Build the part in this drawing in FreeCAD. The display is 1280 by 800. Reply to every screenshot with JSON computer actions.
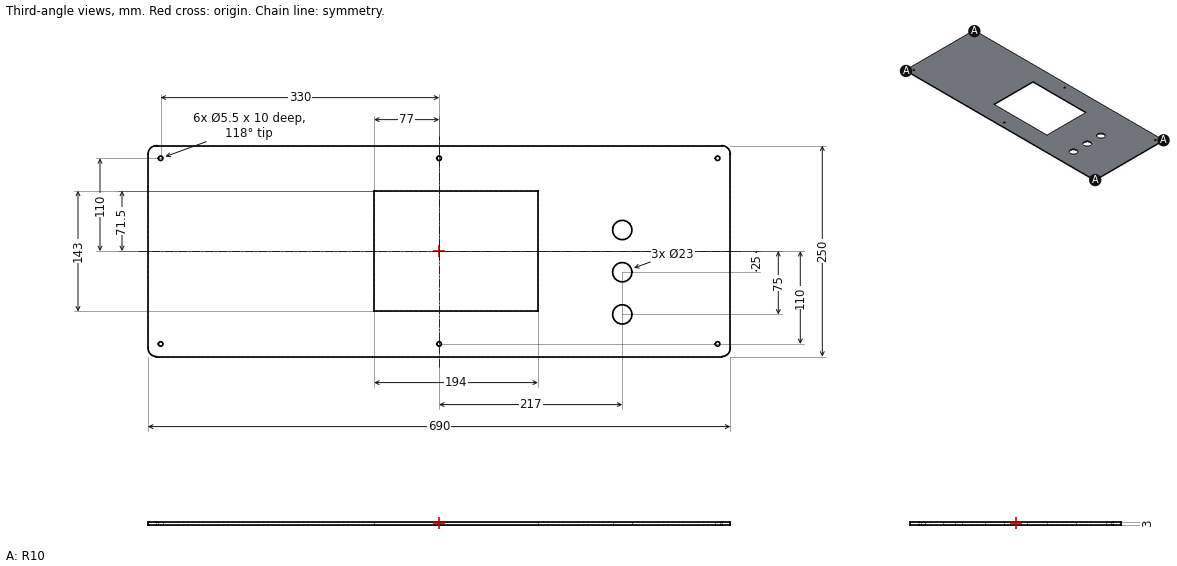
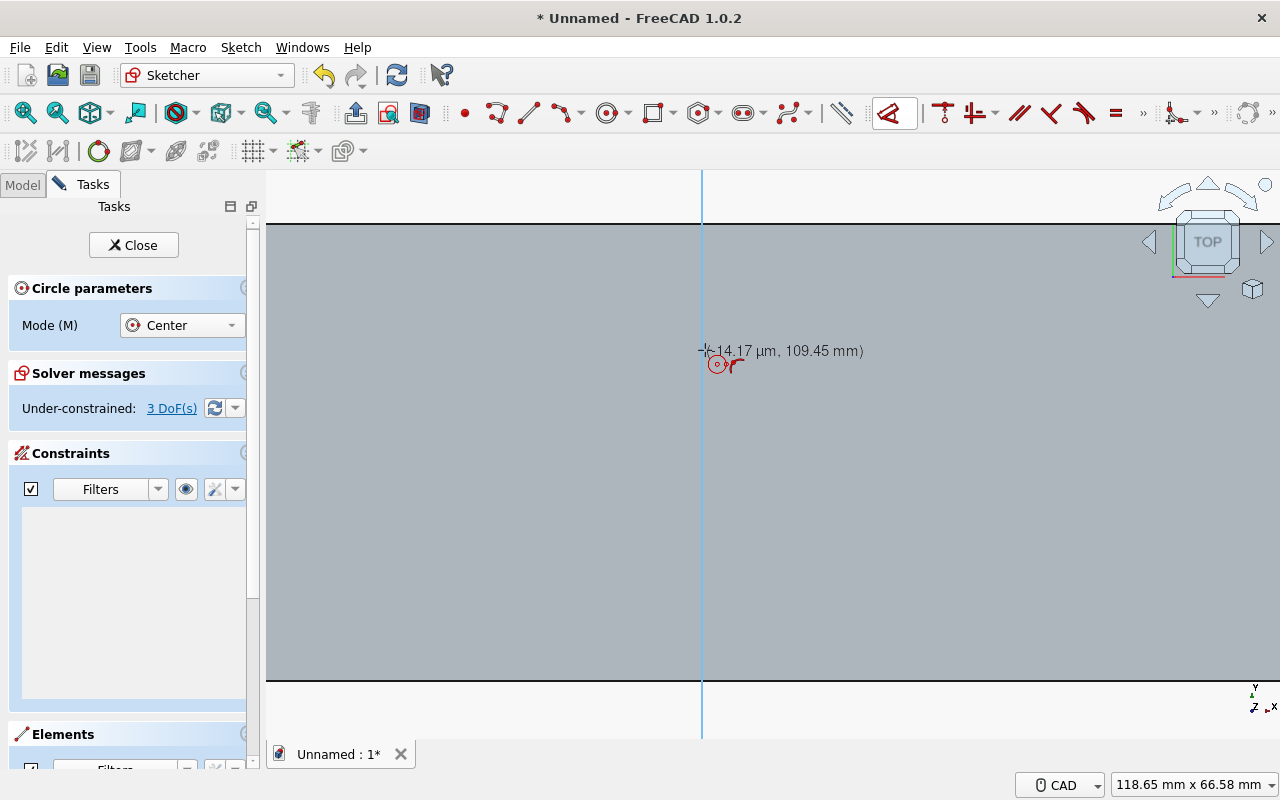
{"action": "scroll", "coordinate": [705, 350], "scroll_direction": "down", "scroll_amount": 11}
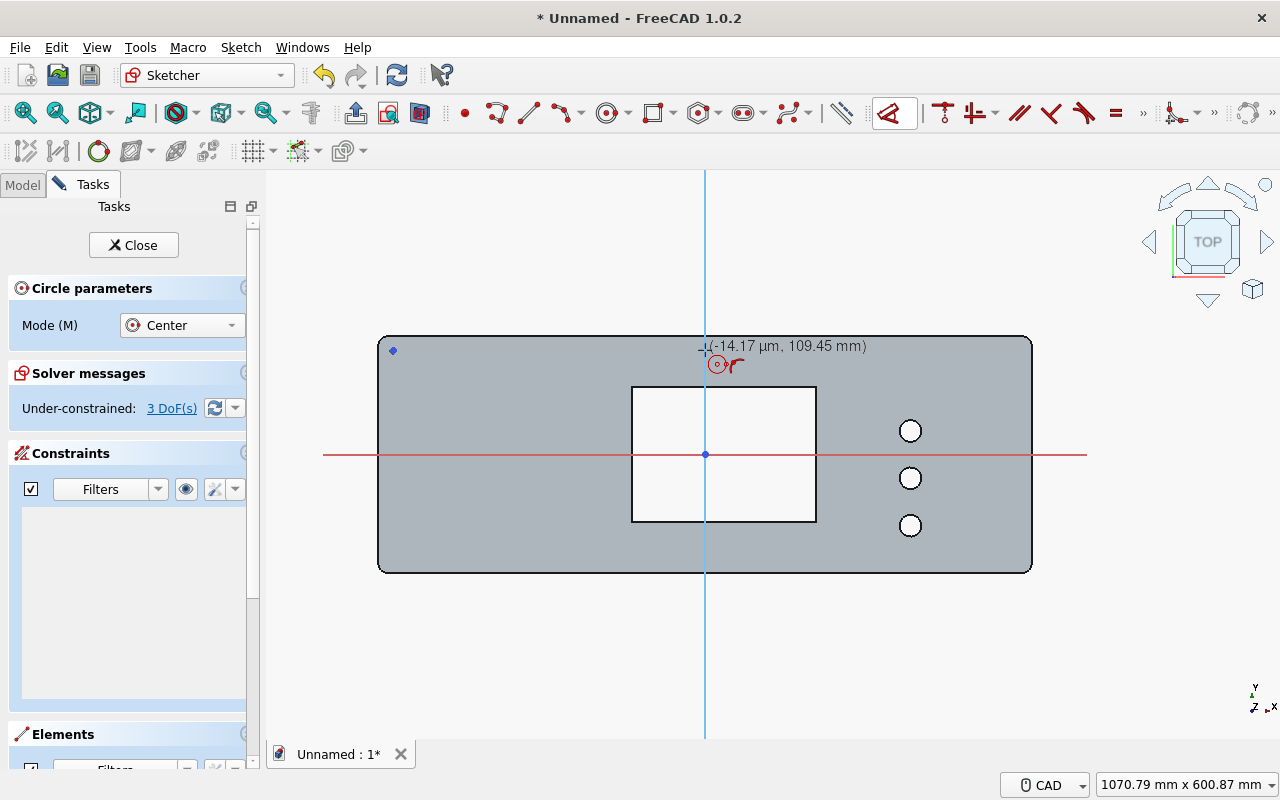
{"action": "left_click", "coordinate": [705, 350]}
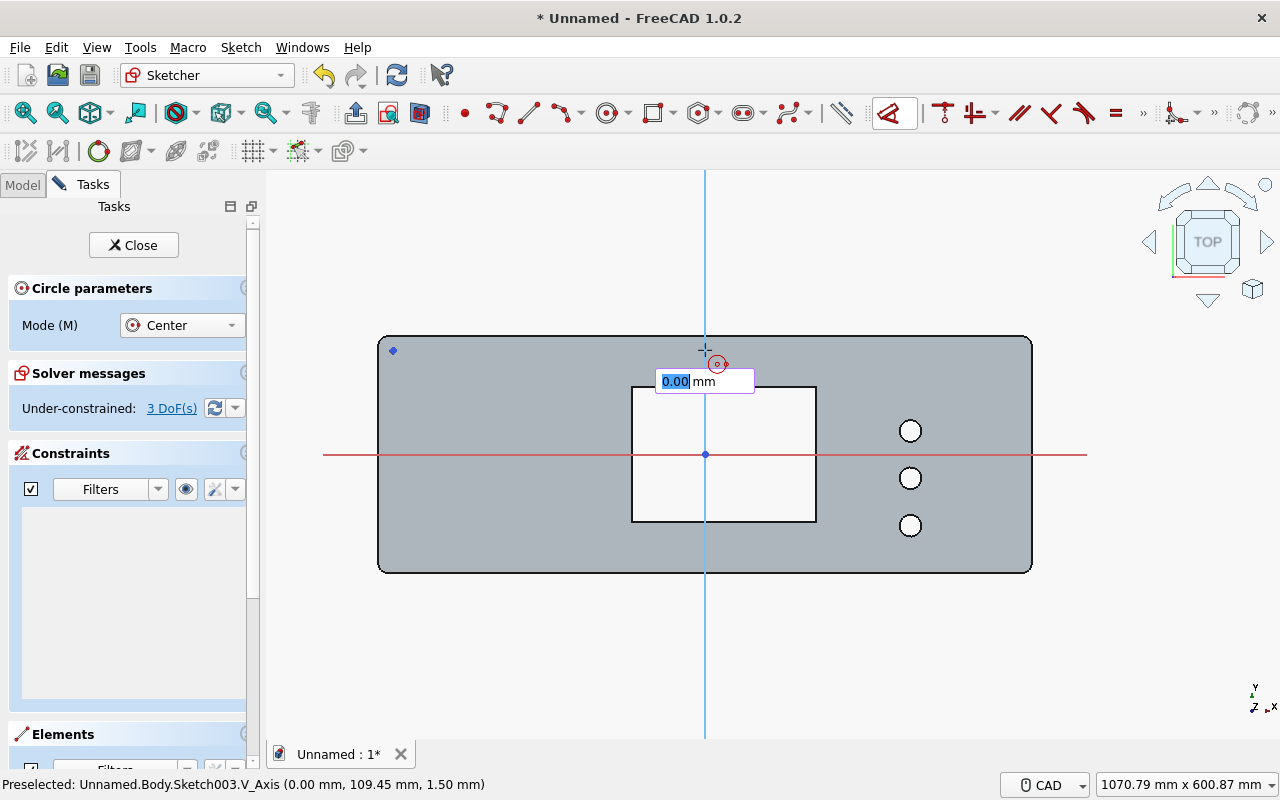
{"action": "scroll", "coordinate": [707, 350], "scroll_direction": "up", "scroll_amount": 10}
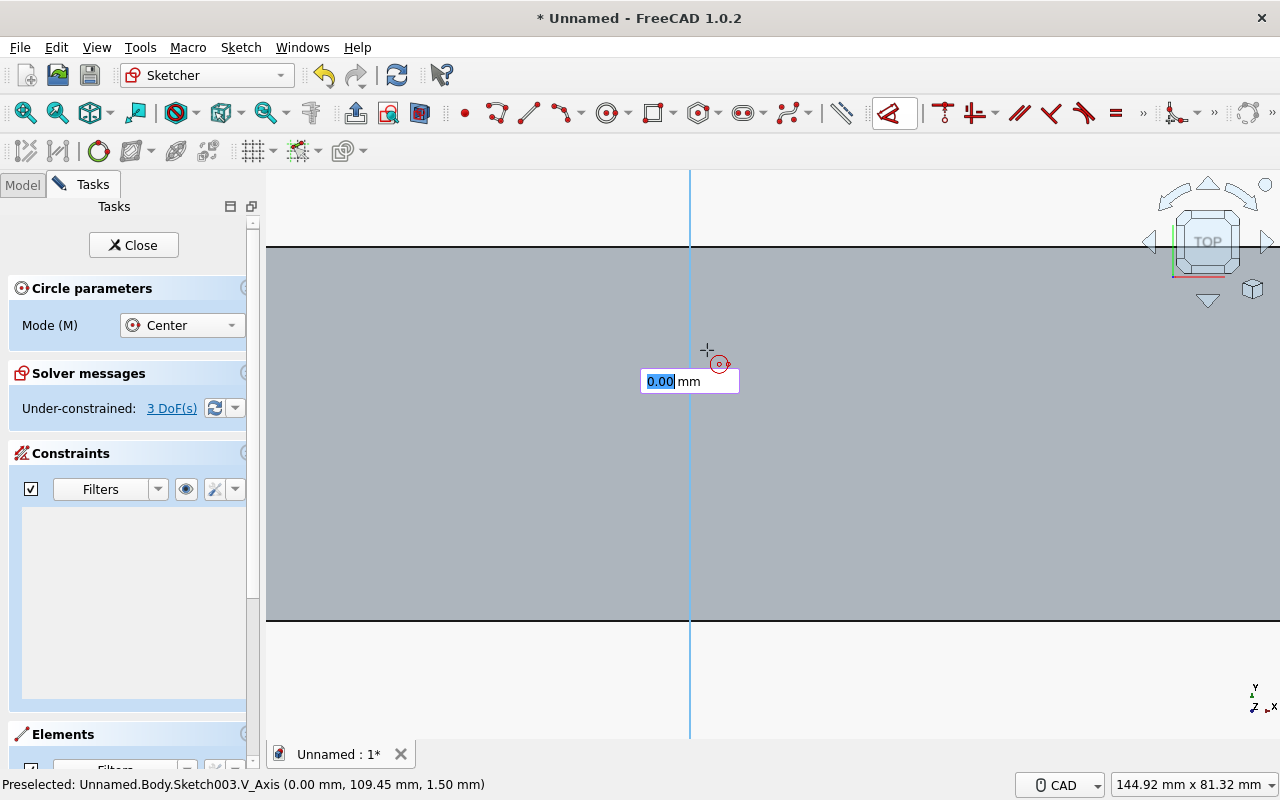
{"action": "left_click", "coordinate": [708, 345]}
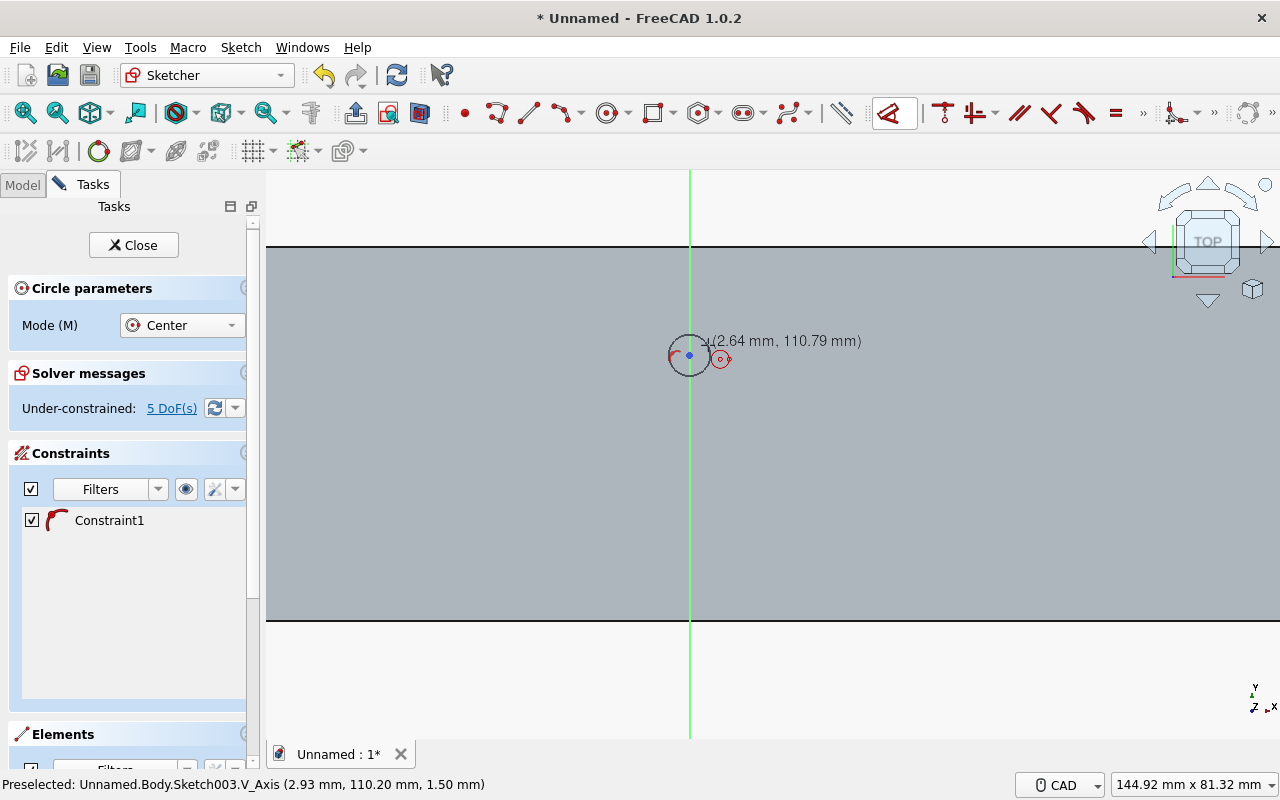
{"action": "scroll", "coordinate": [707, 350], "scroll_direction": "down", "scroll_amount": 10}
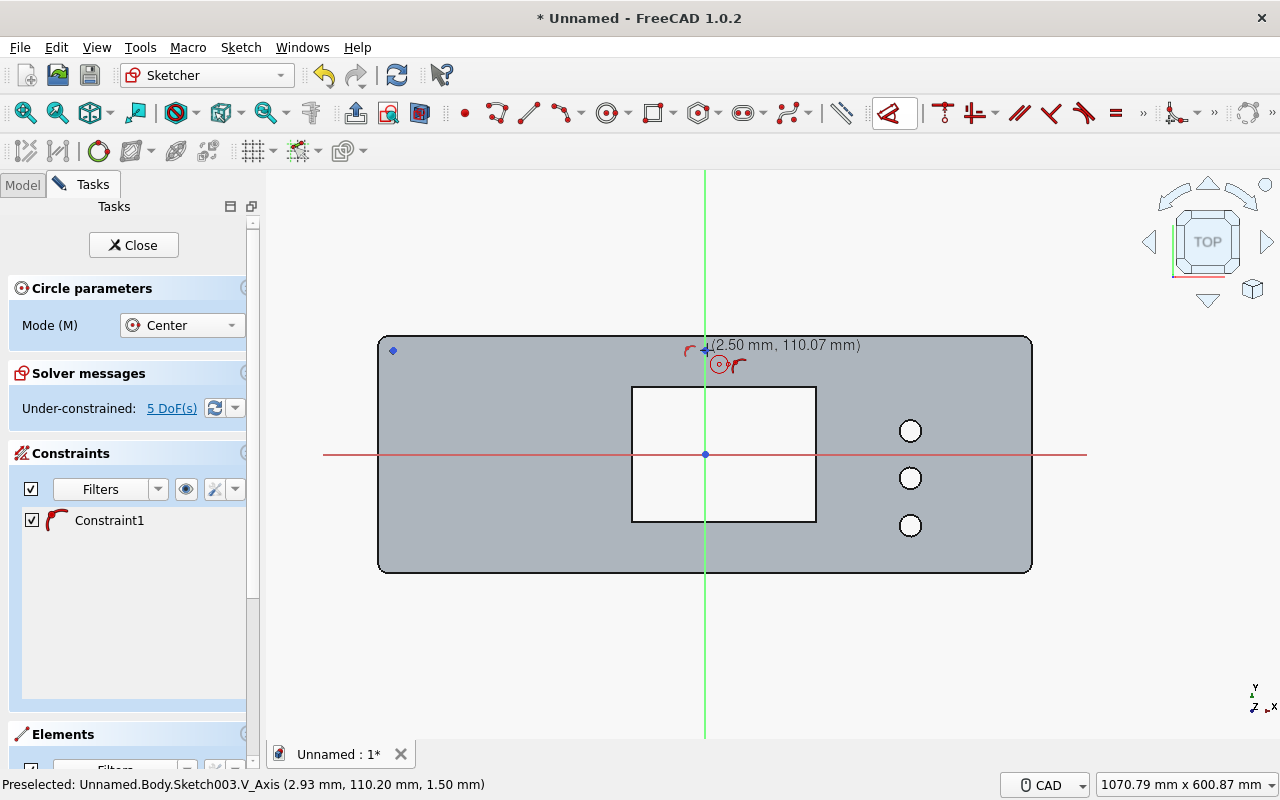
{"action": "scroll", "coordinate": [1018, 350], "scroll_direction": "up", "scroll_amount": 11}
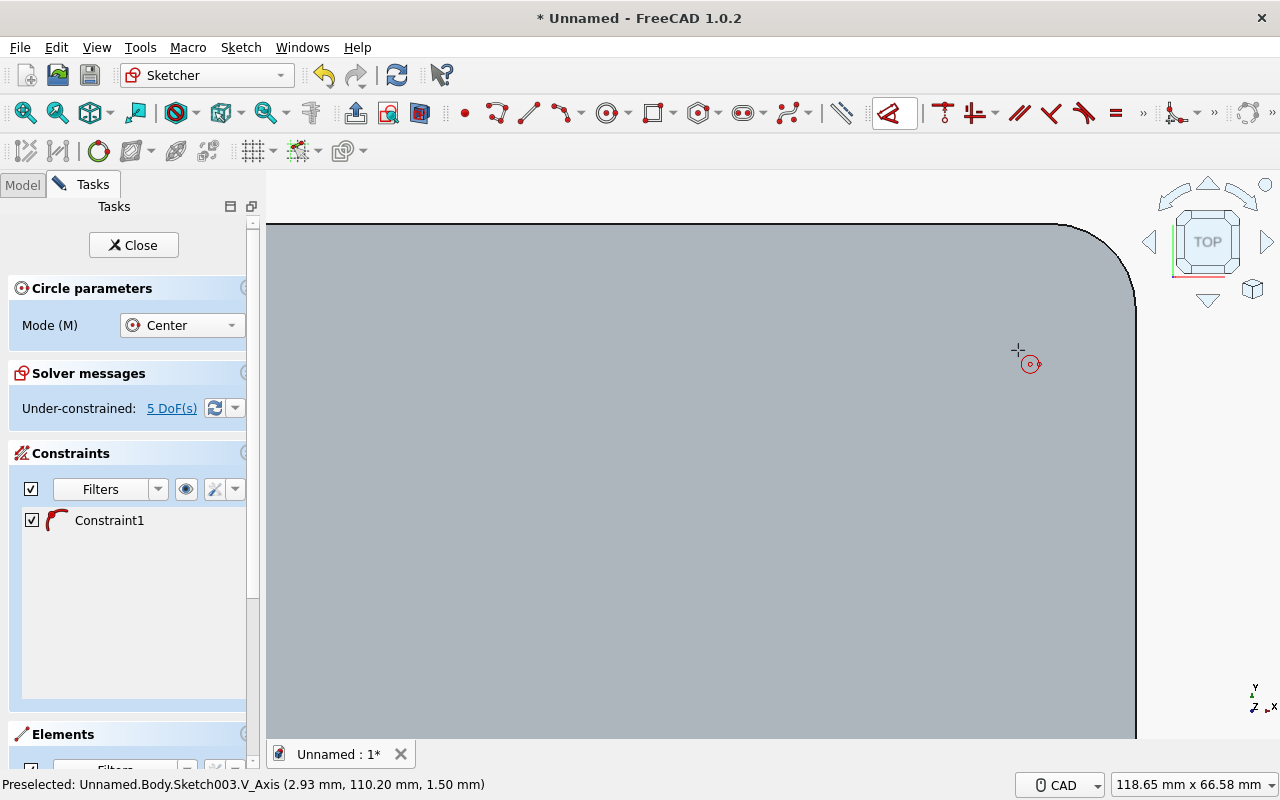
{"action": "scroll", "coordinate": [1018, 350], "scroll_direction": "down", "scroll_amount": 11}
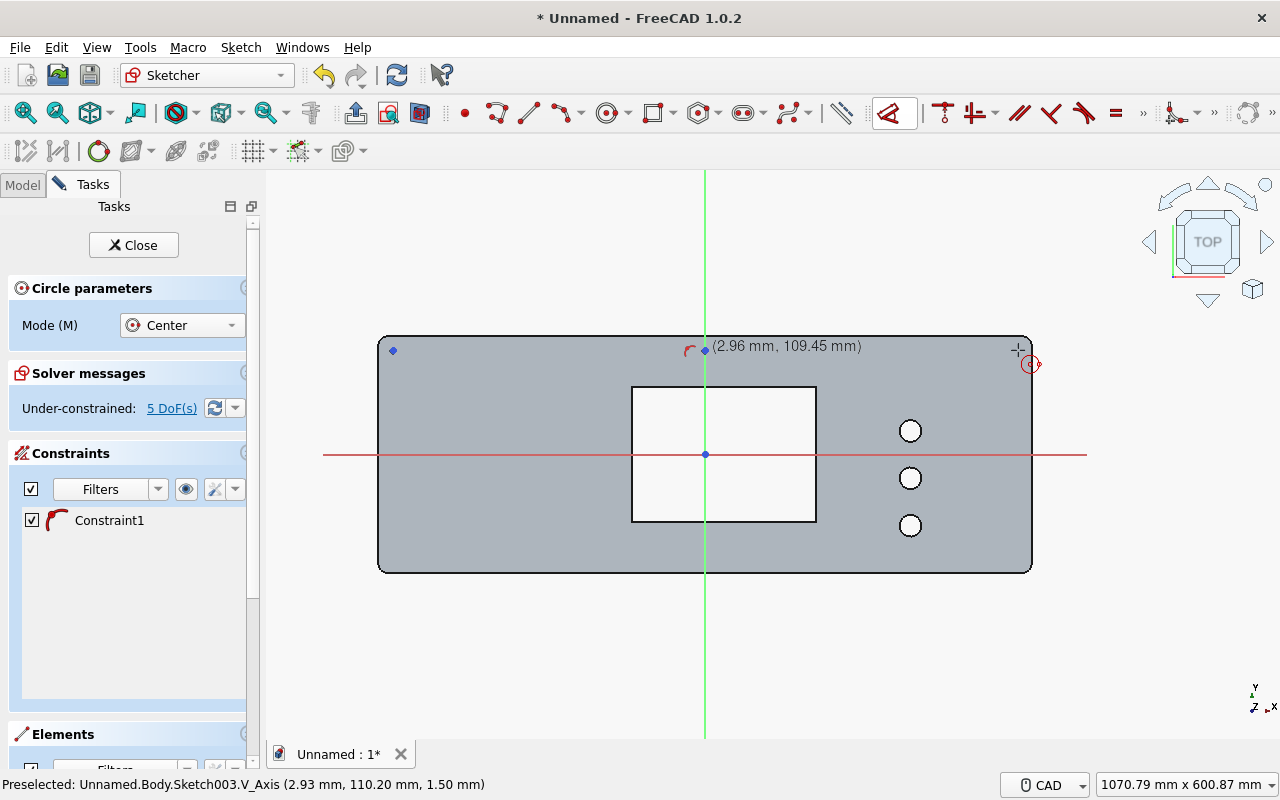
{"action": "left_click", "coordinate": [1018, 350]}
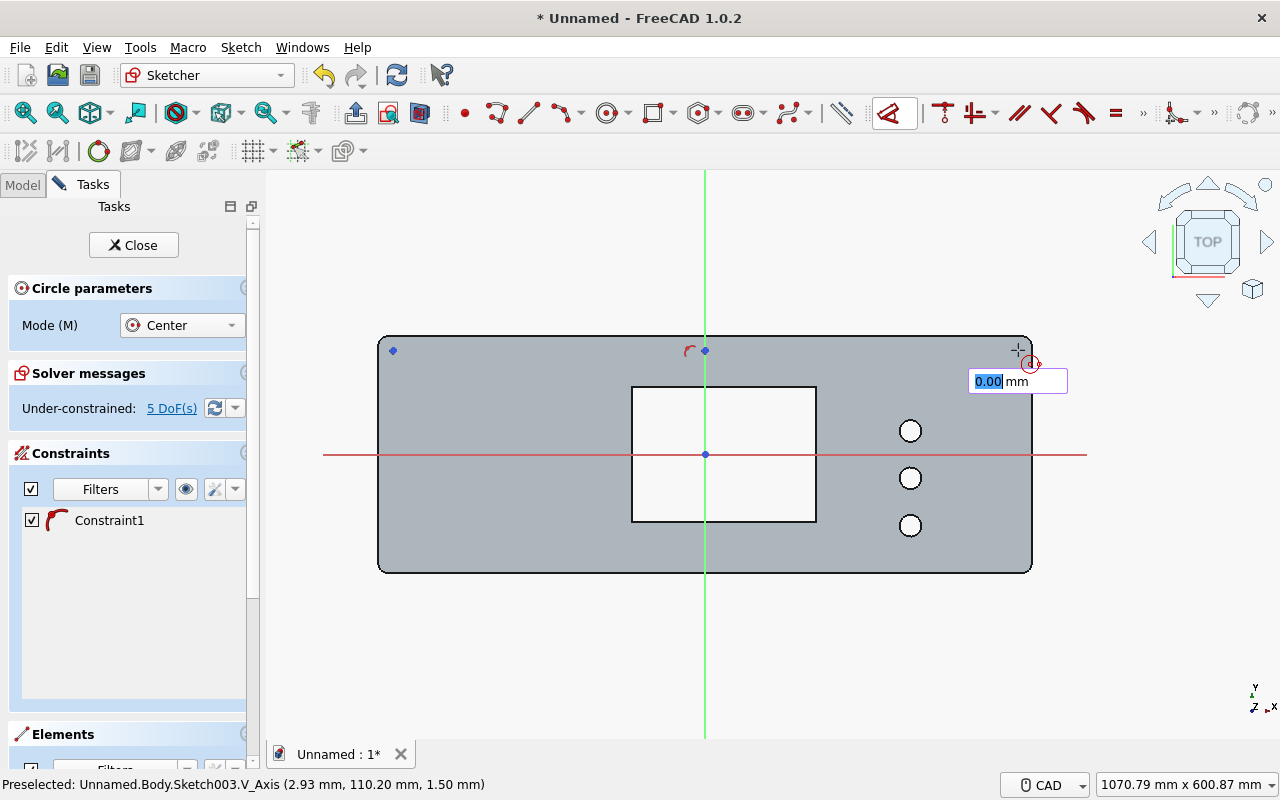
{"action": "scroll", "coordinate": [1019, 349], "scroll_direction": "up", "scroll_amount": 10}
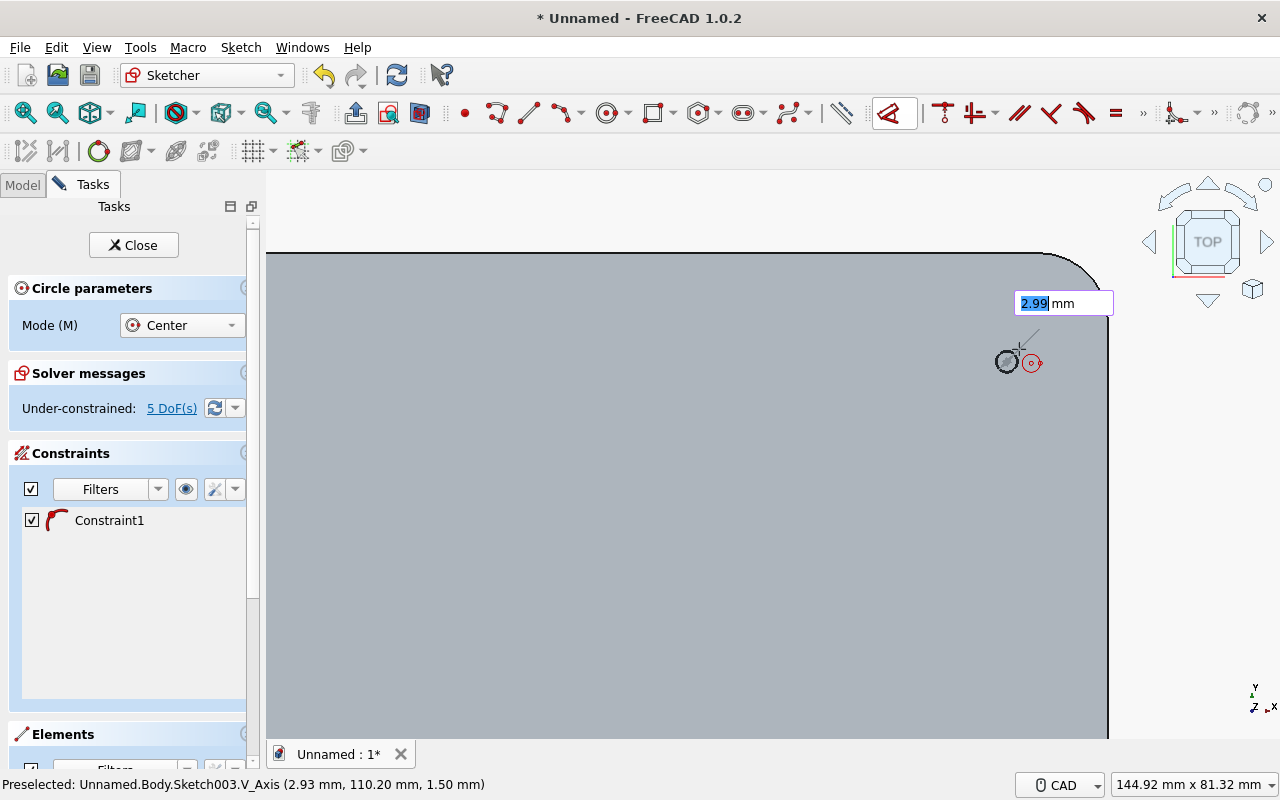
{"action": "left_click", "coordinate": [1017, 344]}